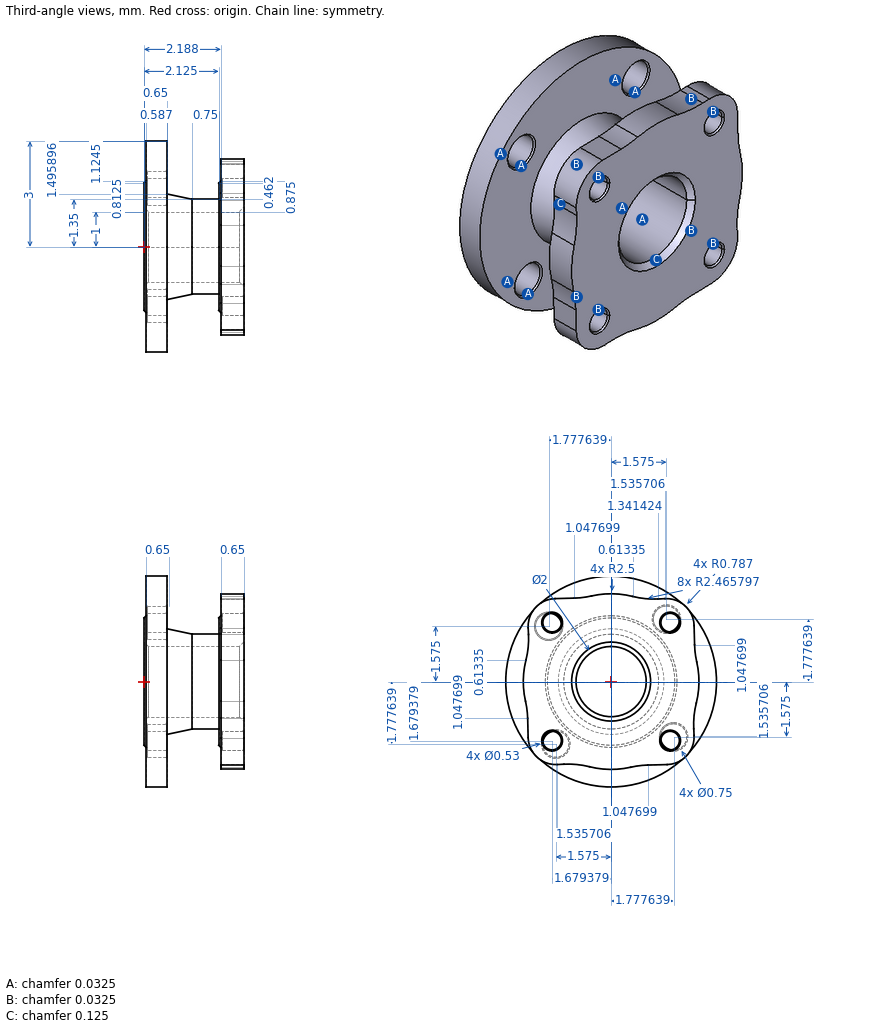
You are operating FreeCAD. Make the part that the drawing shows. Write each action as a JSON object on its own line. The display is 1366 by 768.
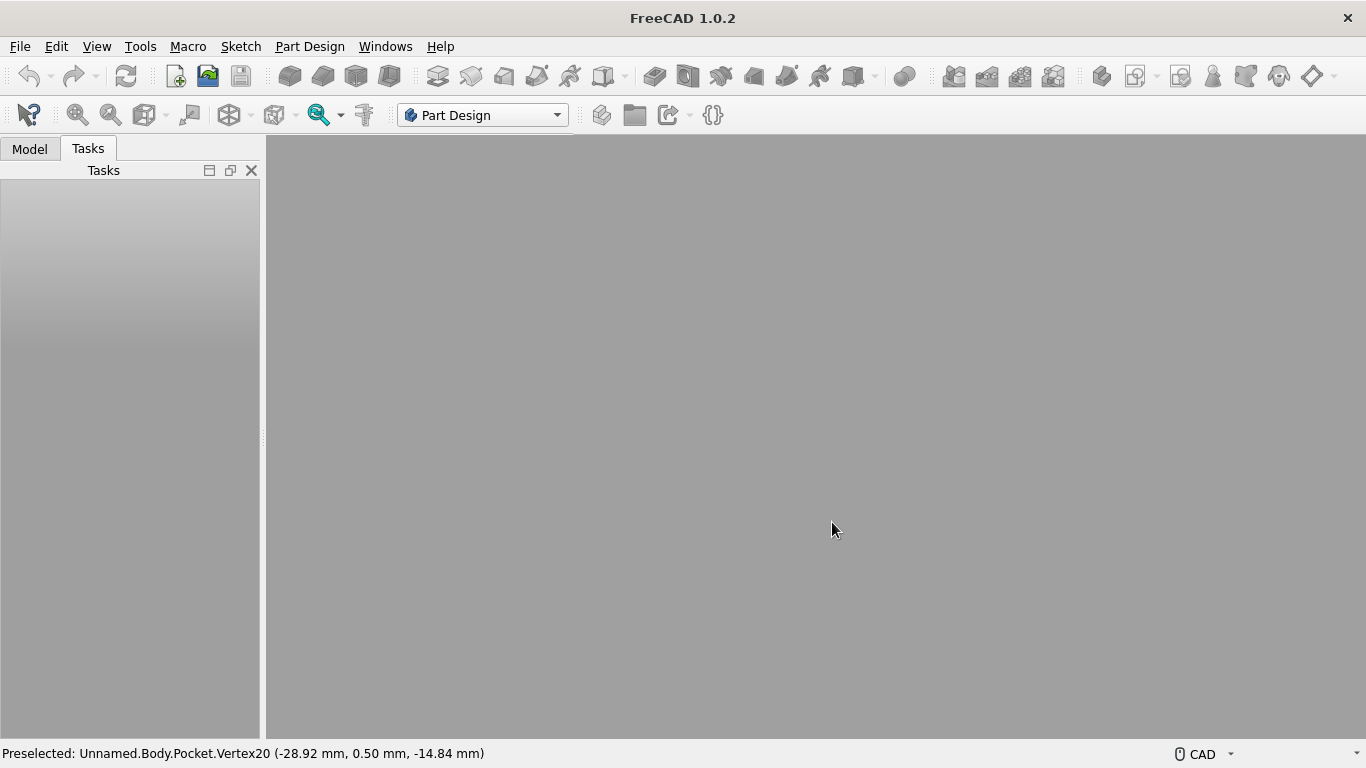
{"action": "left_click", "coordinate": [175, 76]}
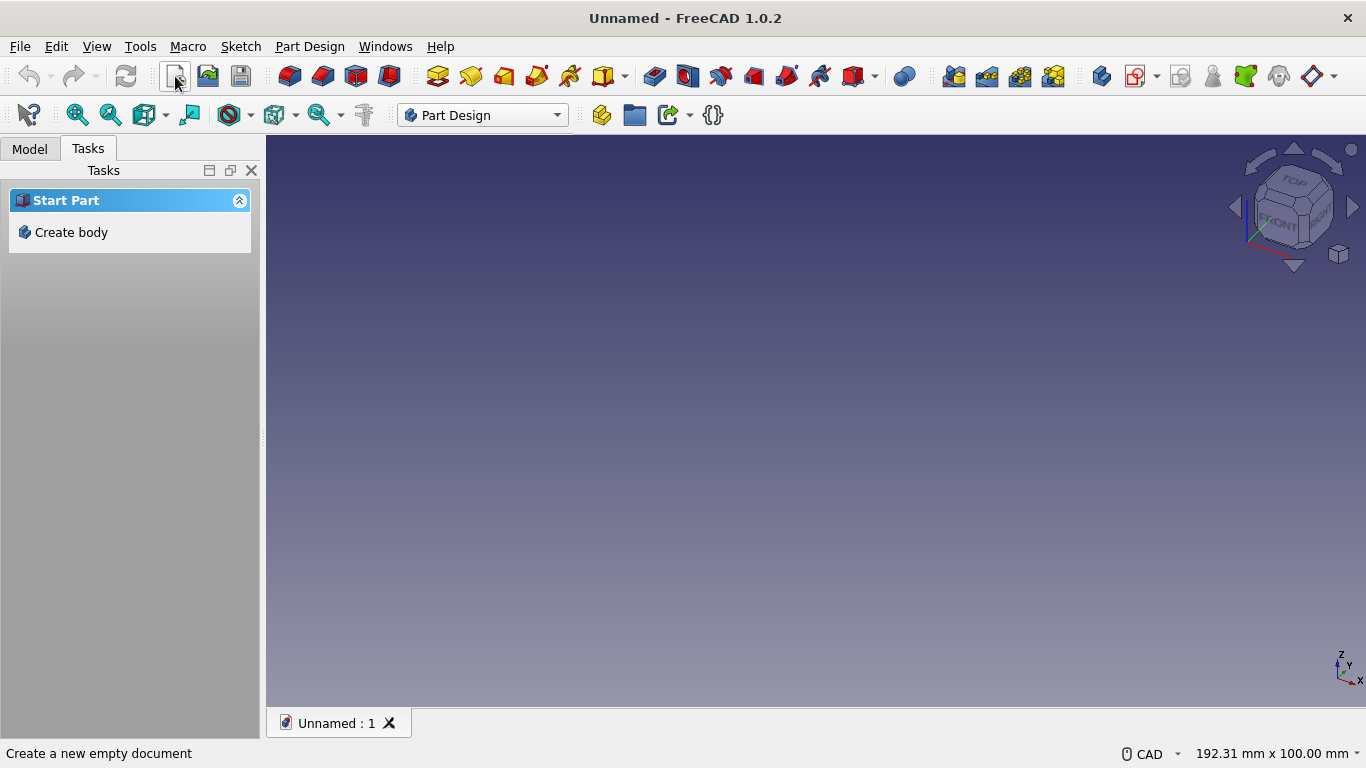
{"action": "left_click", "coordinate": [1134, 76]}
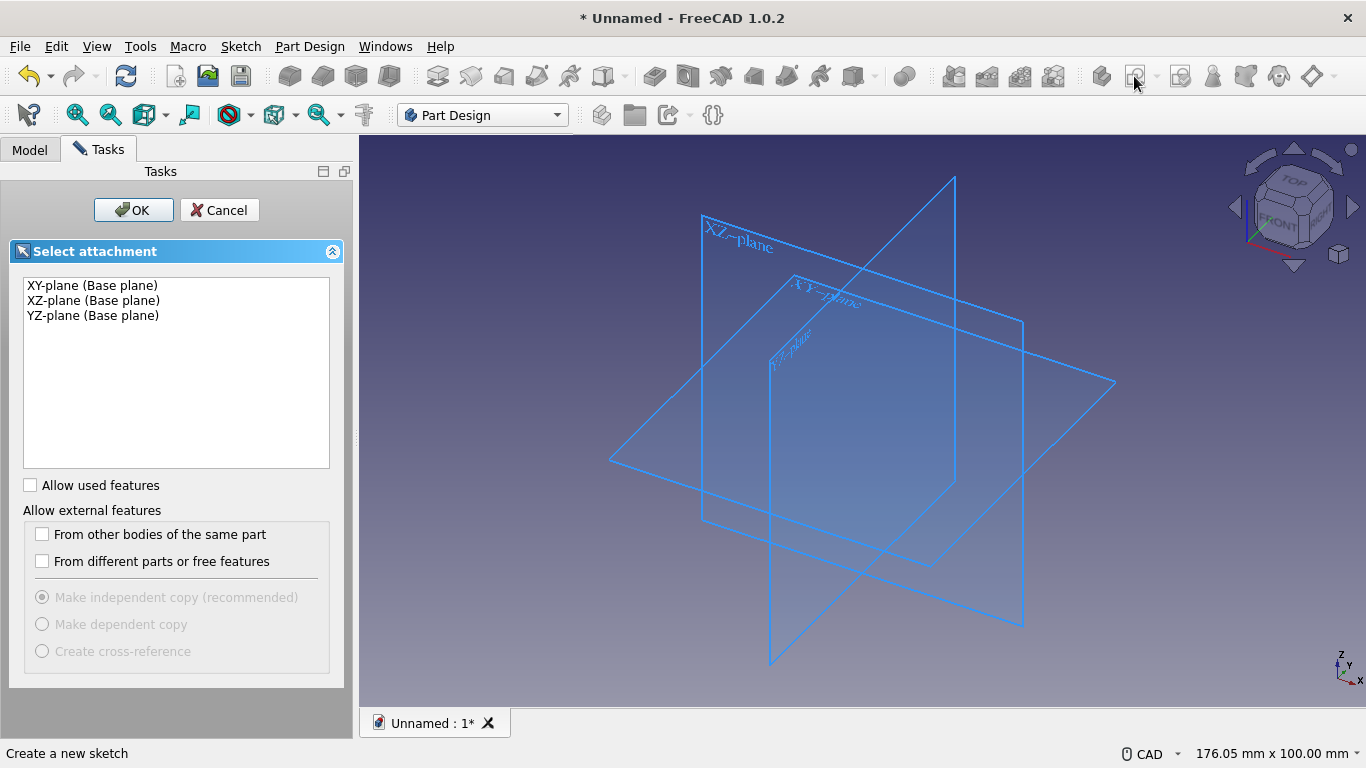
{"action": "left_click", "coordinate": [84, 286]}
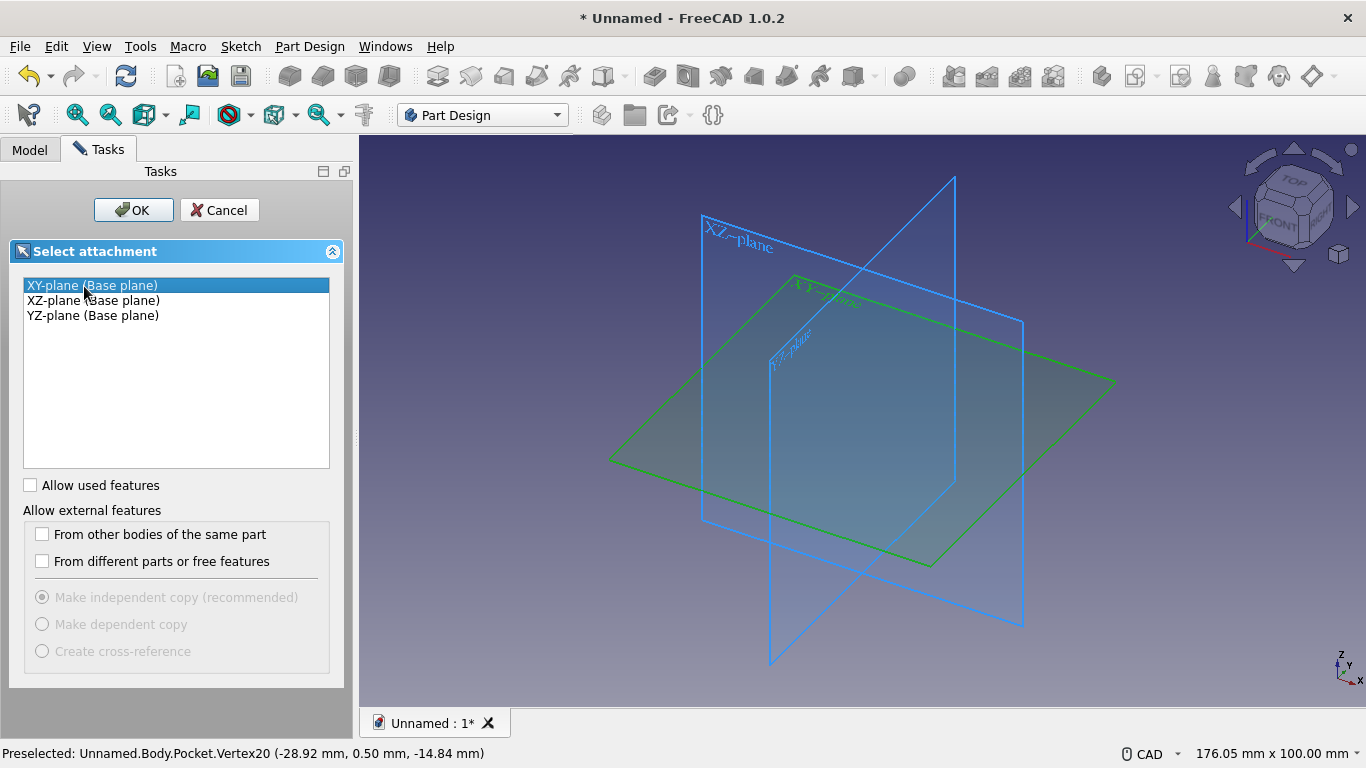
{"action": "left_click", "coordinate": [134, 210]}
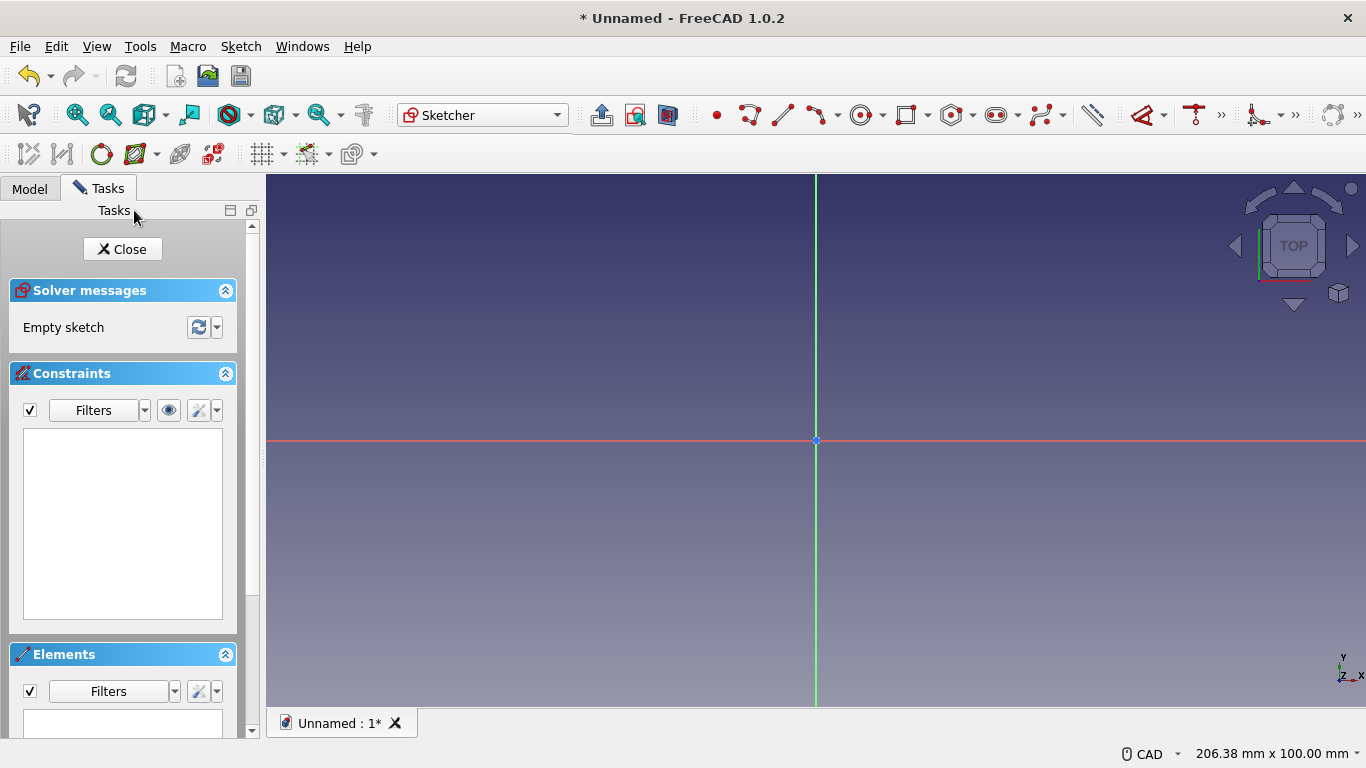
{"action": "scroll", "coordinate": [826, 432], "scroll_direction": "up", "scroll_amount": 15}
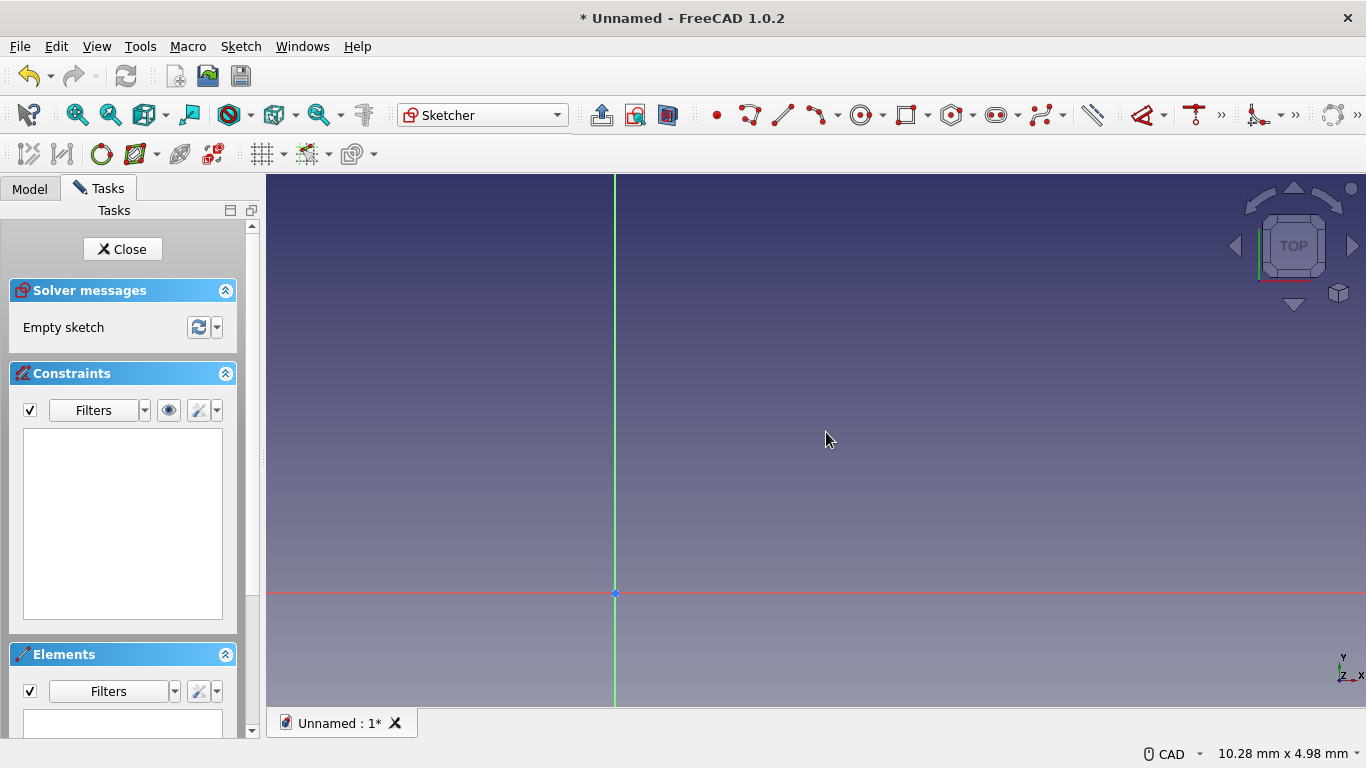
{"action": "left_click", "coordinate": [750, 116]}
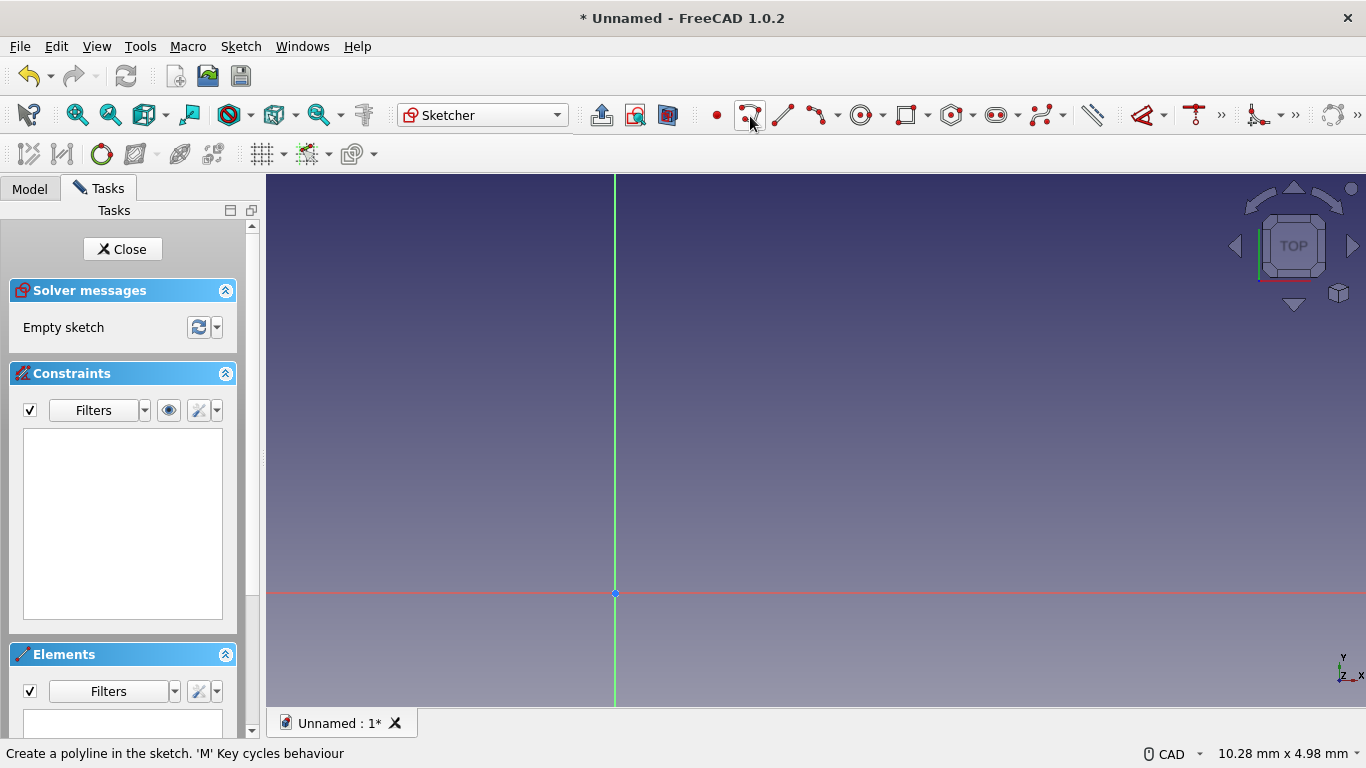
{"action": "left_click", "coordinate": [615, 486]}
{"action": "left_click", "coordinate": [850, 486]}
{"action": "left_click", "coordinate": [850, 393]}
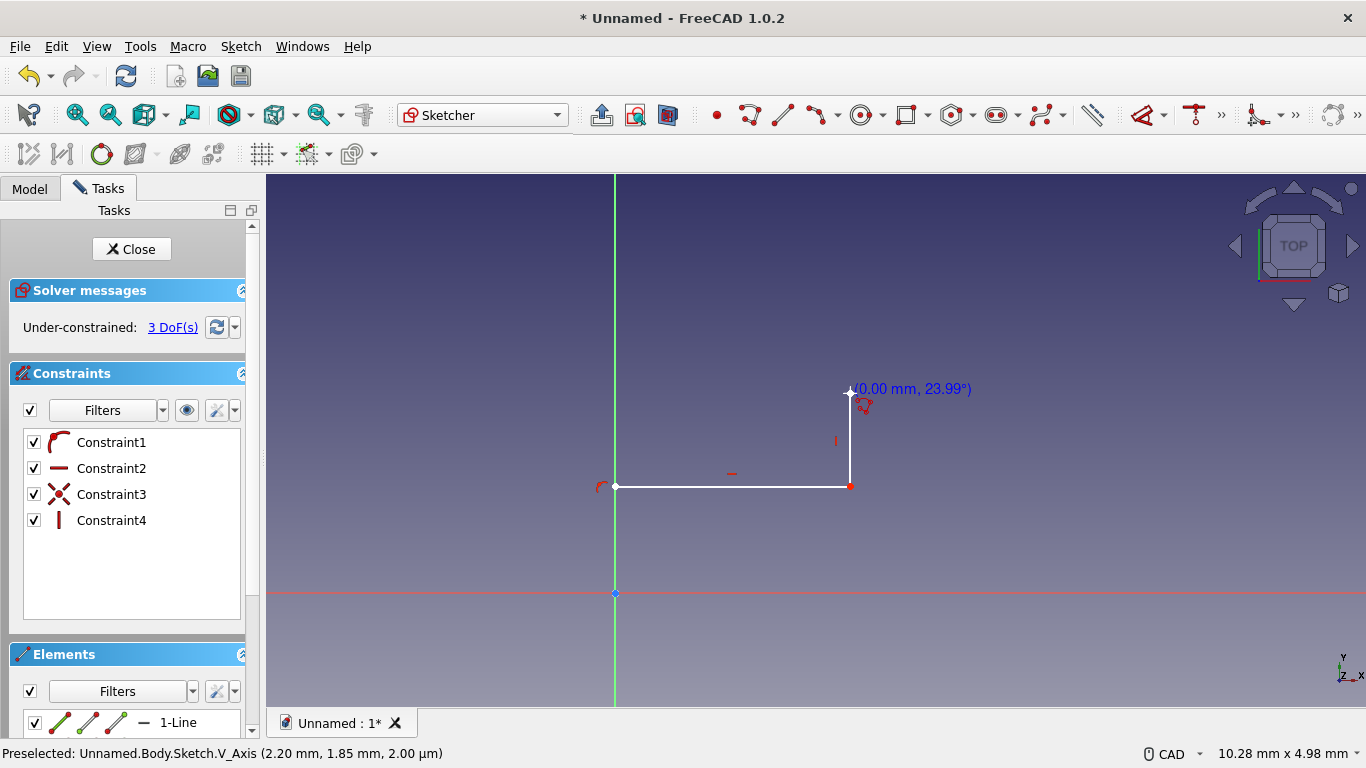
{"action": "scroll", "coordinate": [843, 399], "scroll_direction": "up", "scroll_amount": 5}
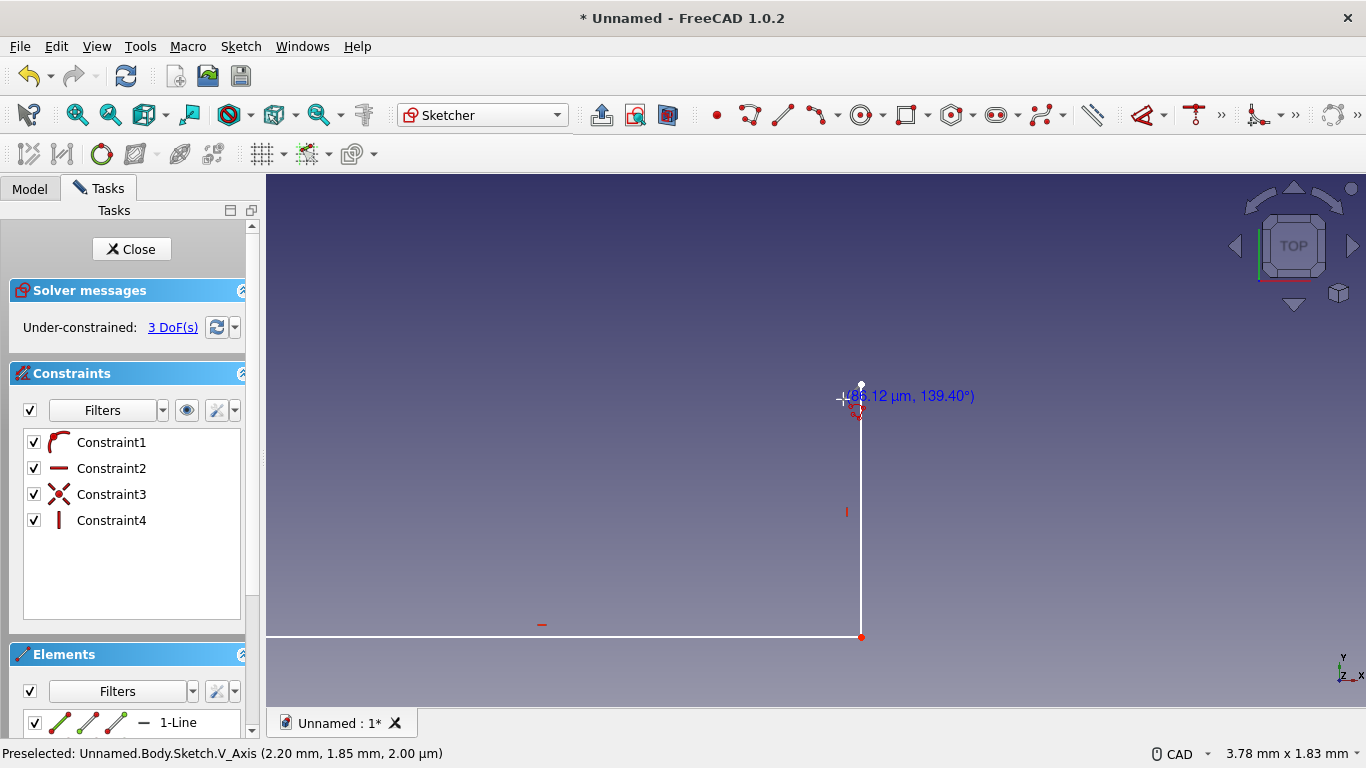
{"action": "left_click", "coordinate": [842, 400]}
{"action": "left_click", "coordinate": [842, 534]}
{"action": "left_click", "coordinate": [624, 534]}
{"action": "left_click", "coordinate": [413, 489]}